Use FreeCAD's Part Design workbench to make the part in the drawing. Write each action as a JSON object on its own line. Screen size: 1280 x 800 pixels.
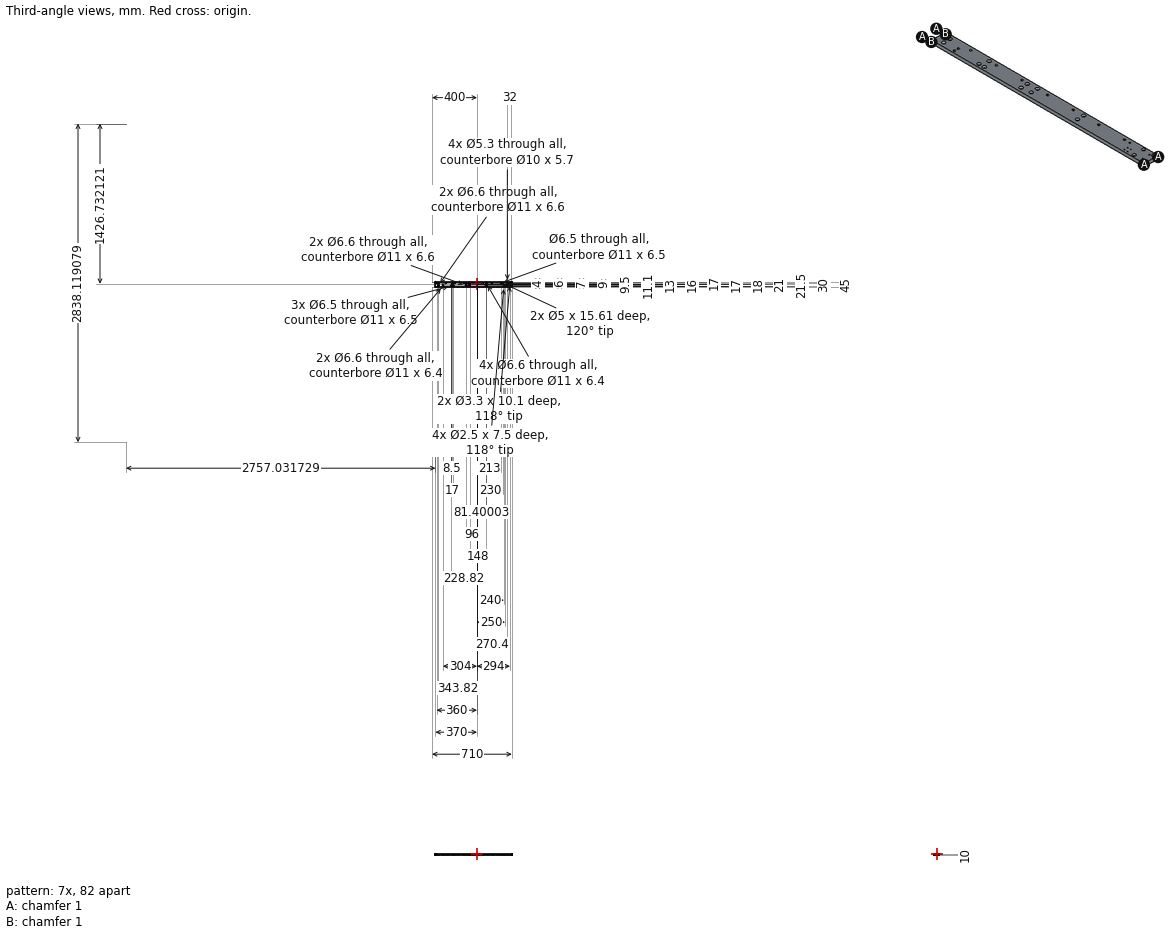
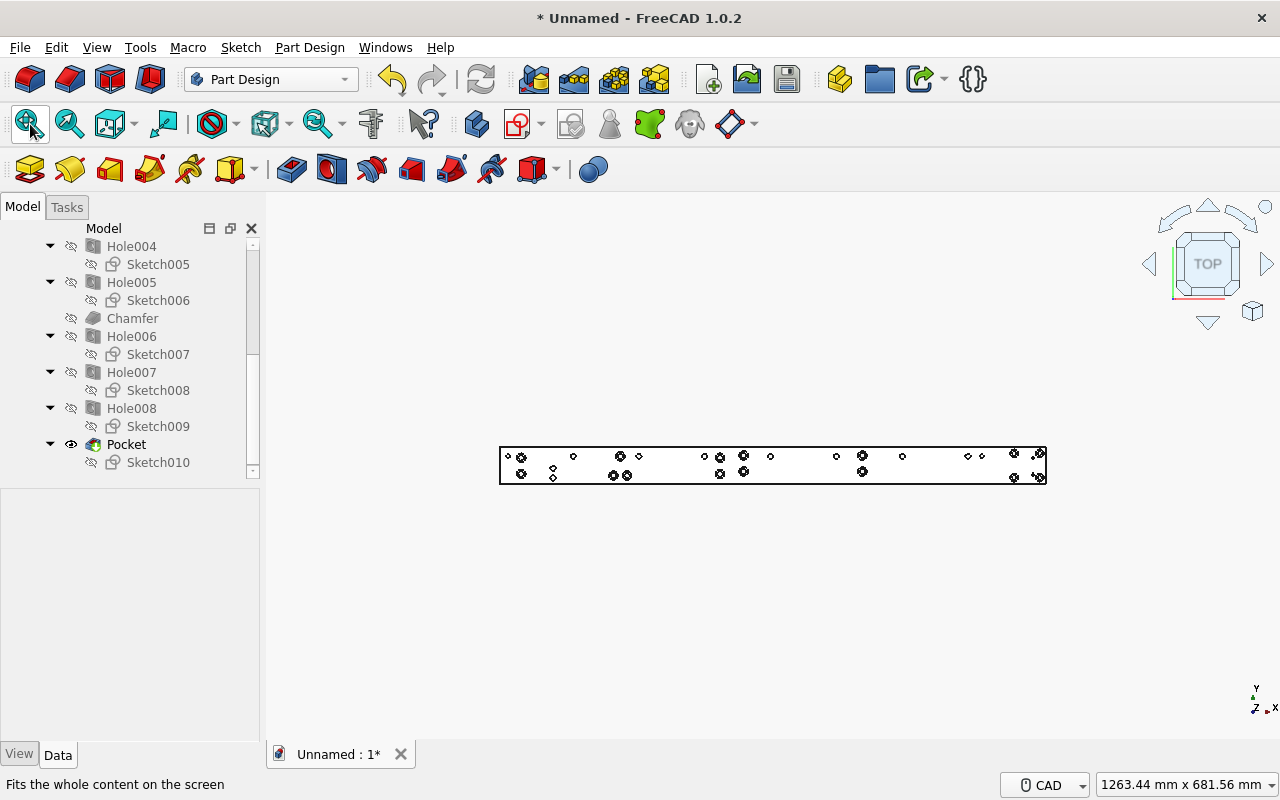
{"action": "scroll", "coordinate": [500, 483], "scroll_direction": "up", "scroll_amount": 9}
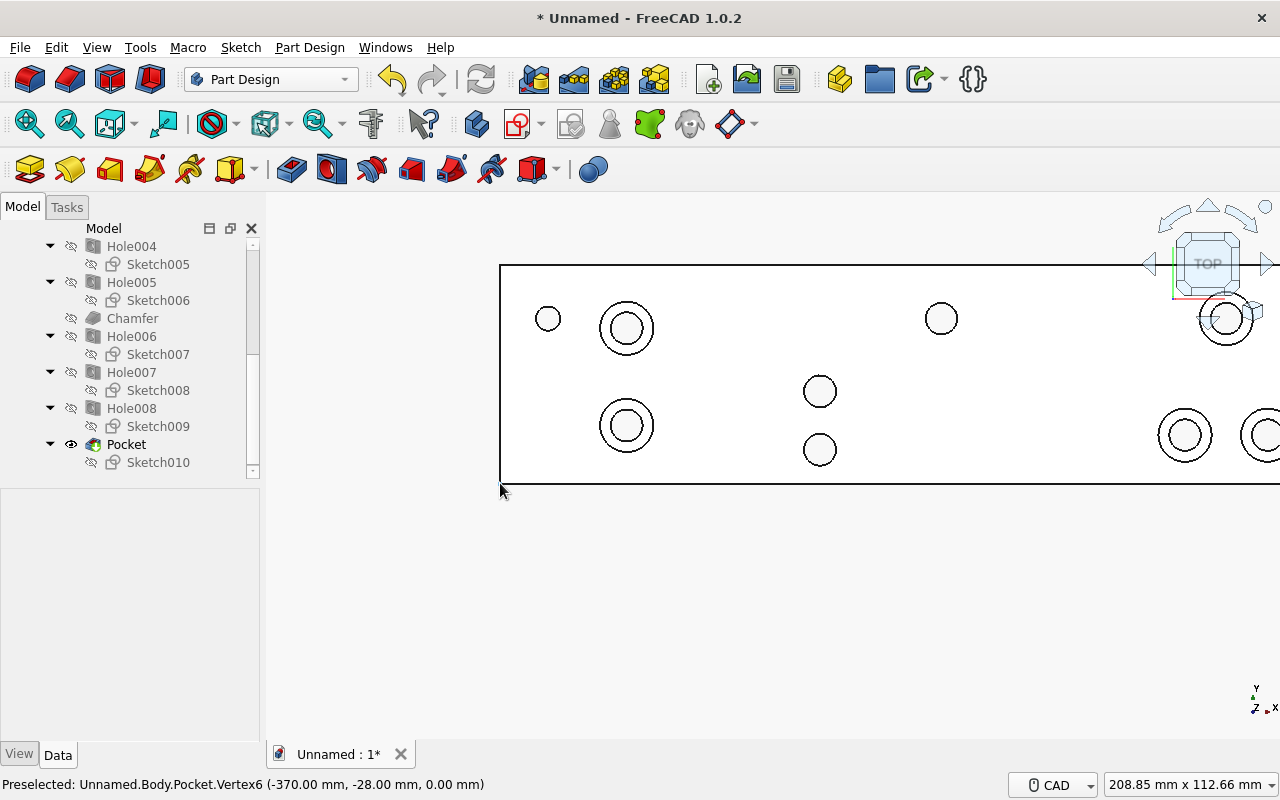
{"action": "left_click", "coordinate": [30, 124]}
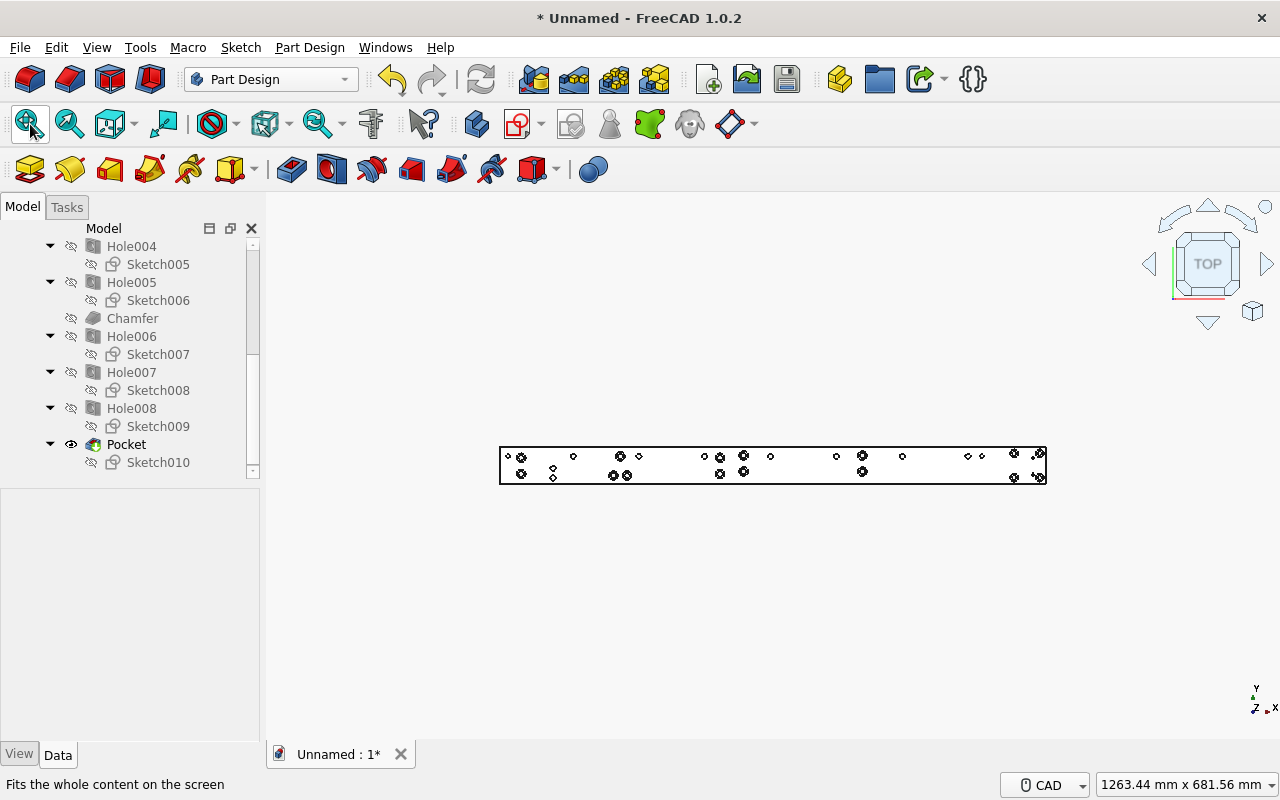
{"action": "key", "text": "0"}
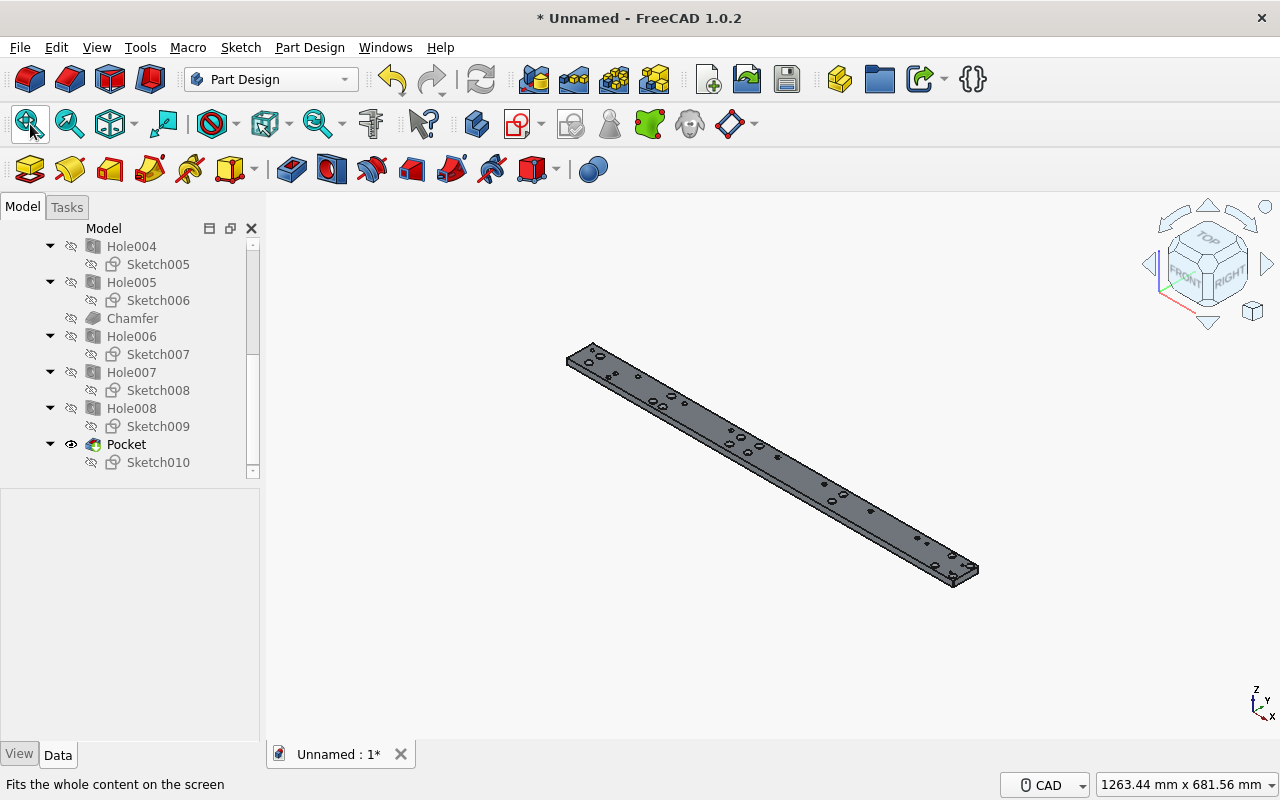
{"action": "left_click", "coordinate": [30, 124]}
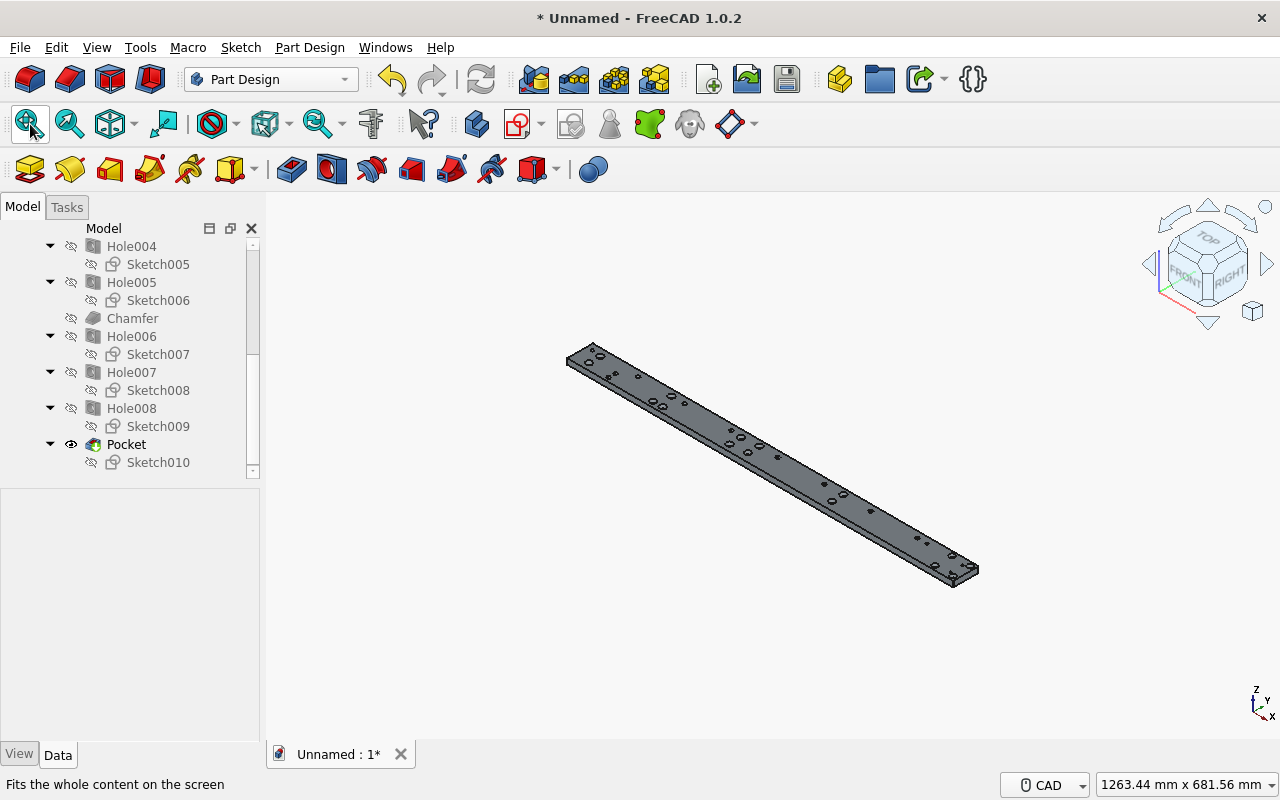
{"action": "scroll", "coordinate": [567, 360], "scroll_direction": "up", "scroll_amount": 9}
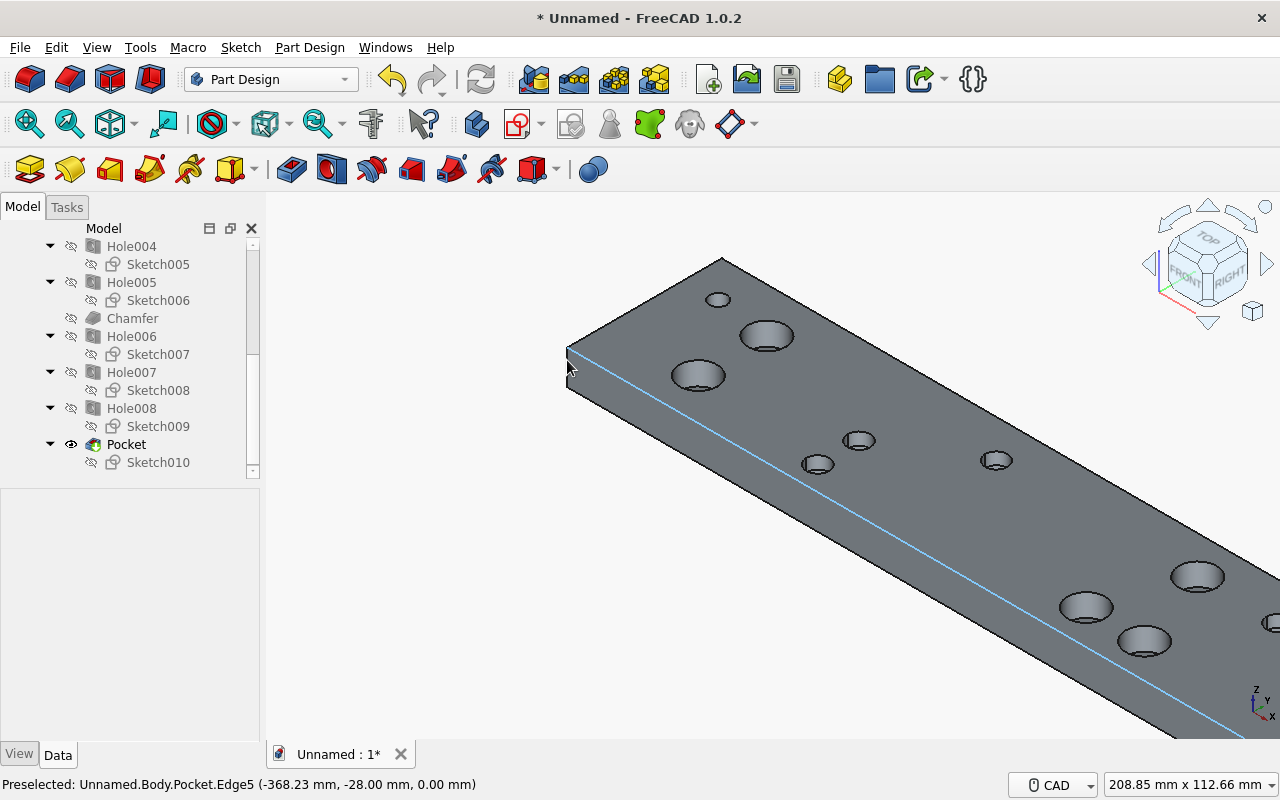
{"action": "left_click", "coordinate": [30, 124]}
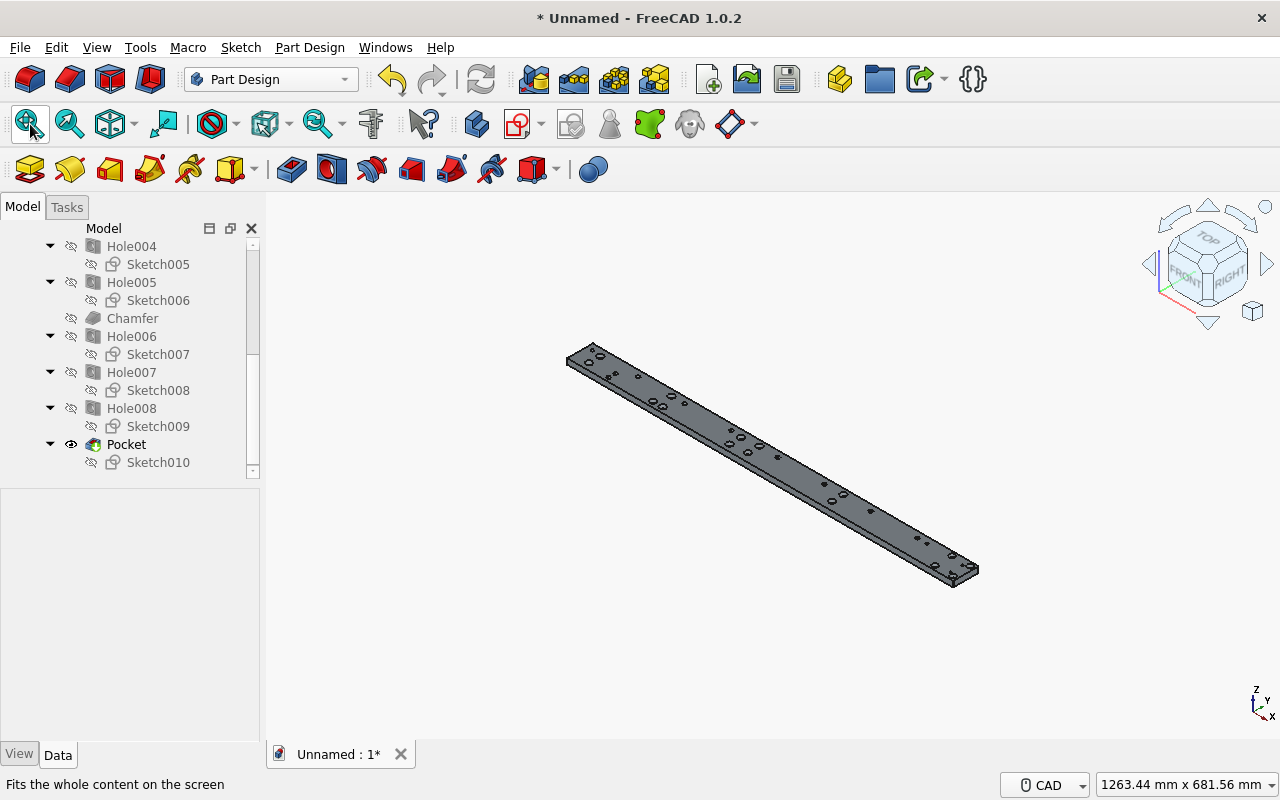
{"action": "key", "text": "1"}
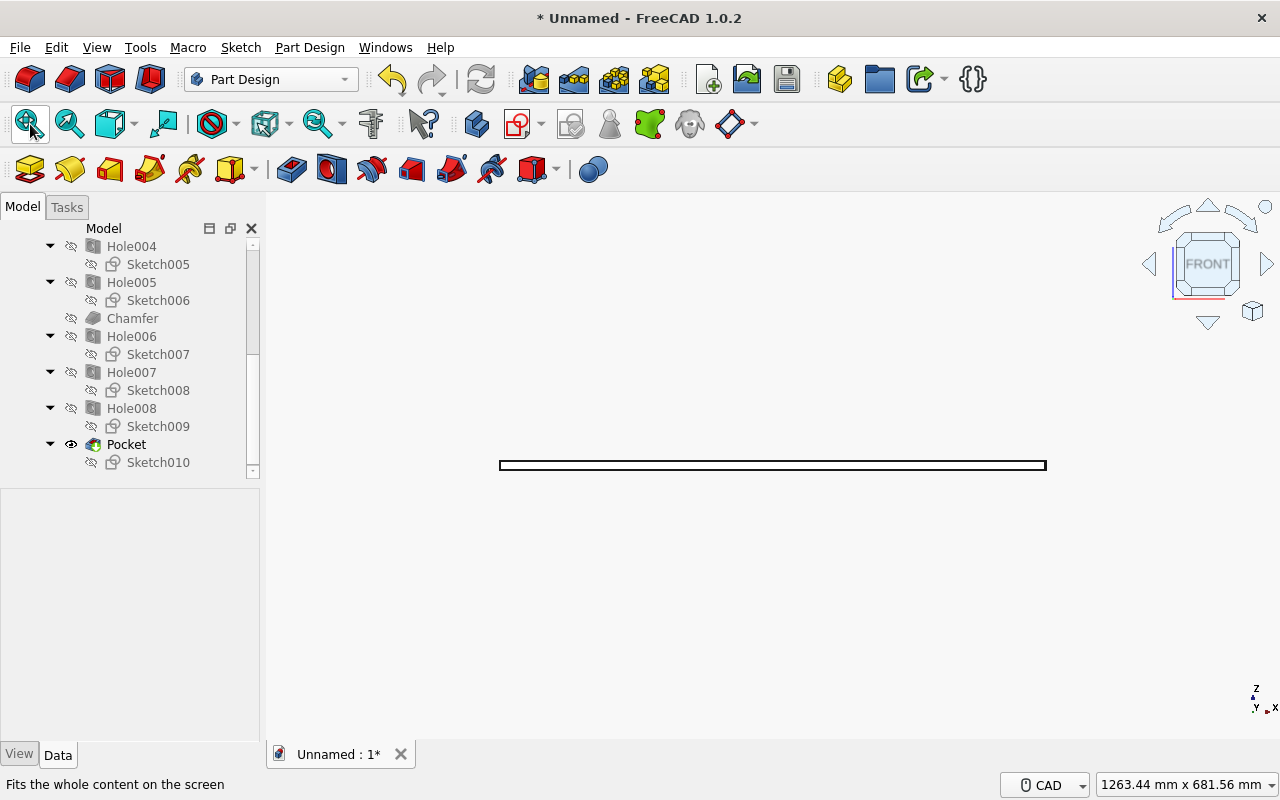
{"action": "scroll", "coordinate": [500, 464], "scroll_direction": "up", "scroll_amount": 9}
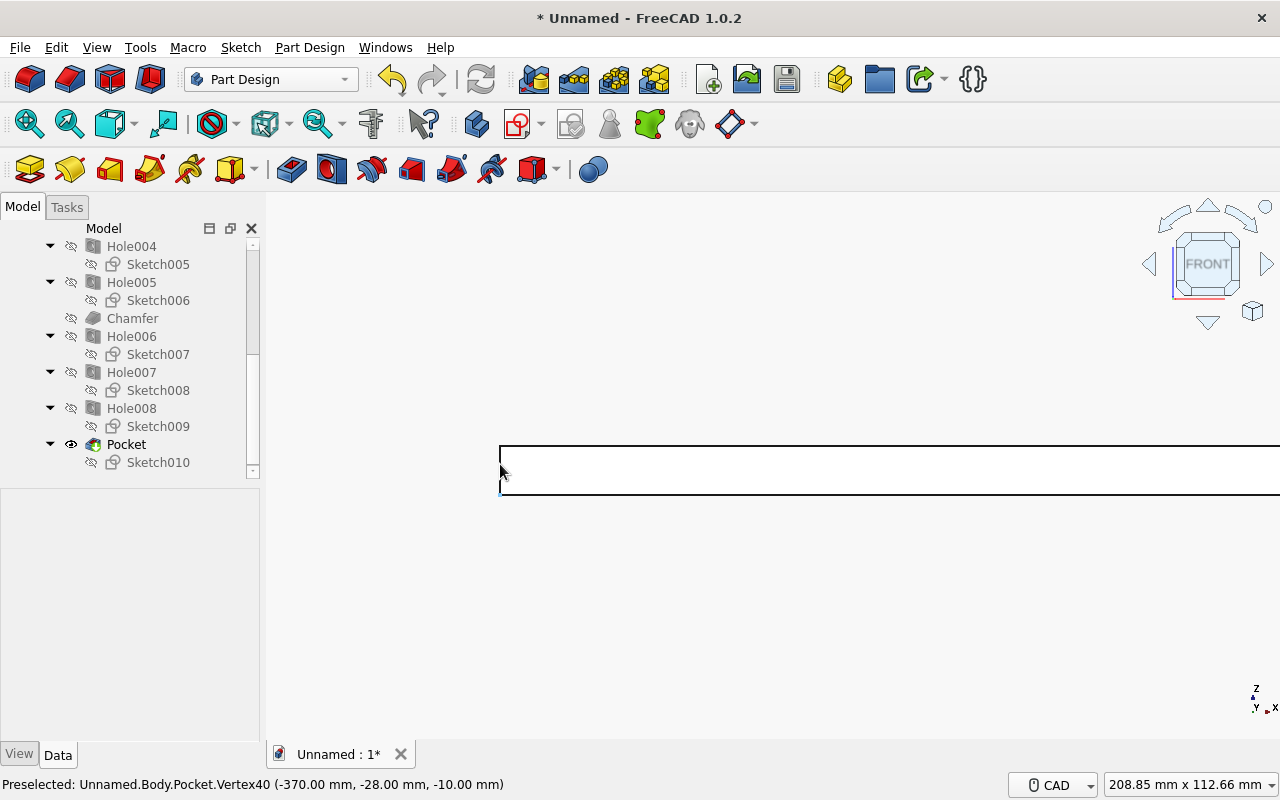
{"action": "left_click", "coordinate": [500, 470]}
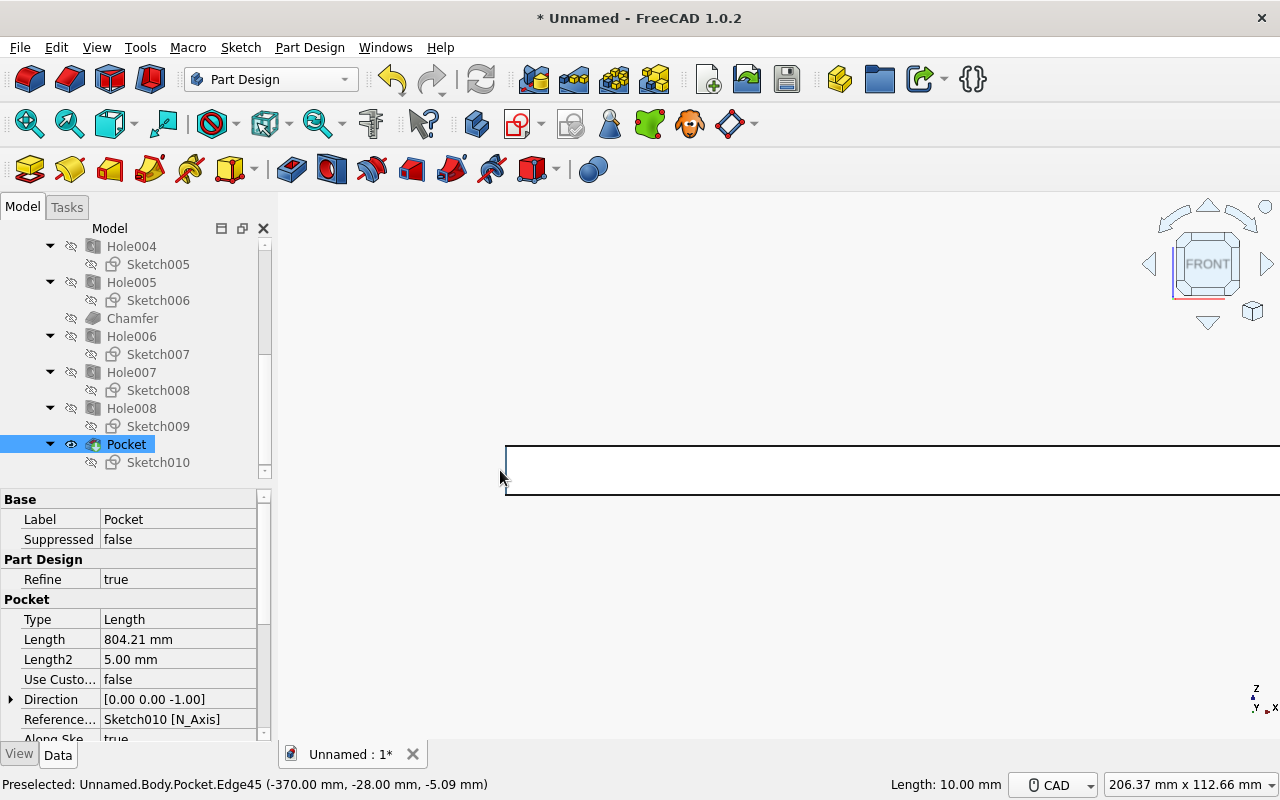
{"action": "left_click", "coordinate": [30, 124]}